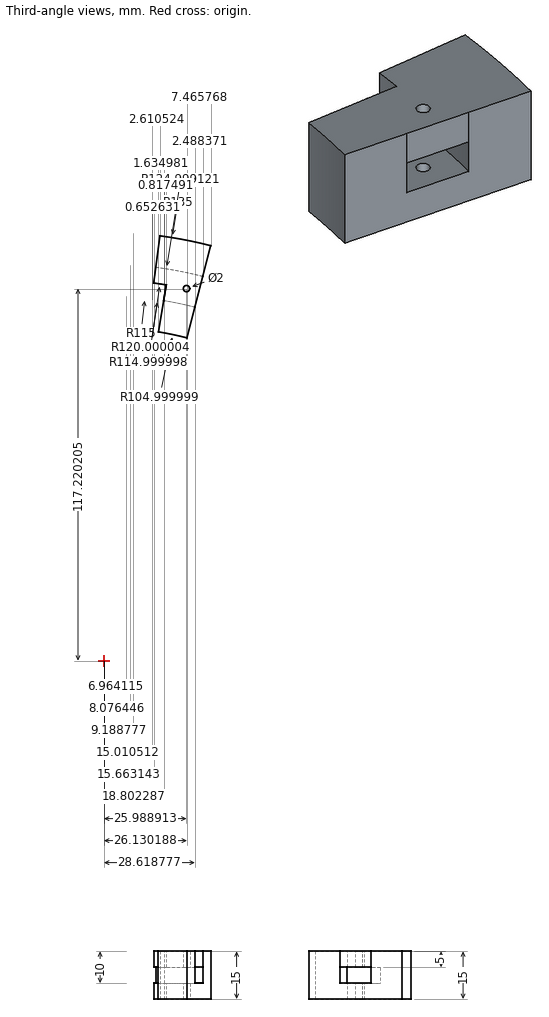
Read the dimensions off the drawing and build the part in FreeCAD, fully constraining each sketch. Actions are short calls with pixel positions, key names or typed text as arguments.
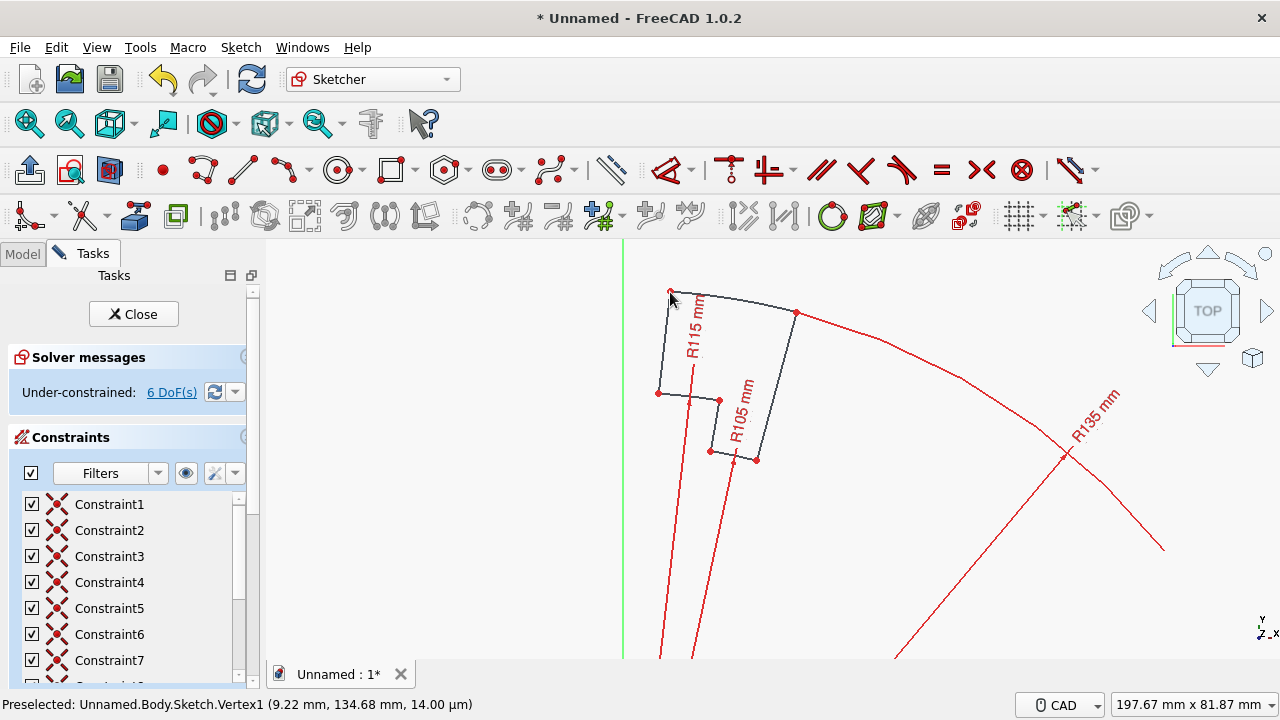
click(670, 292)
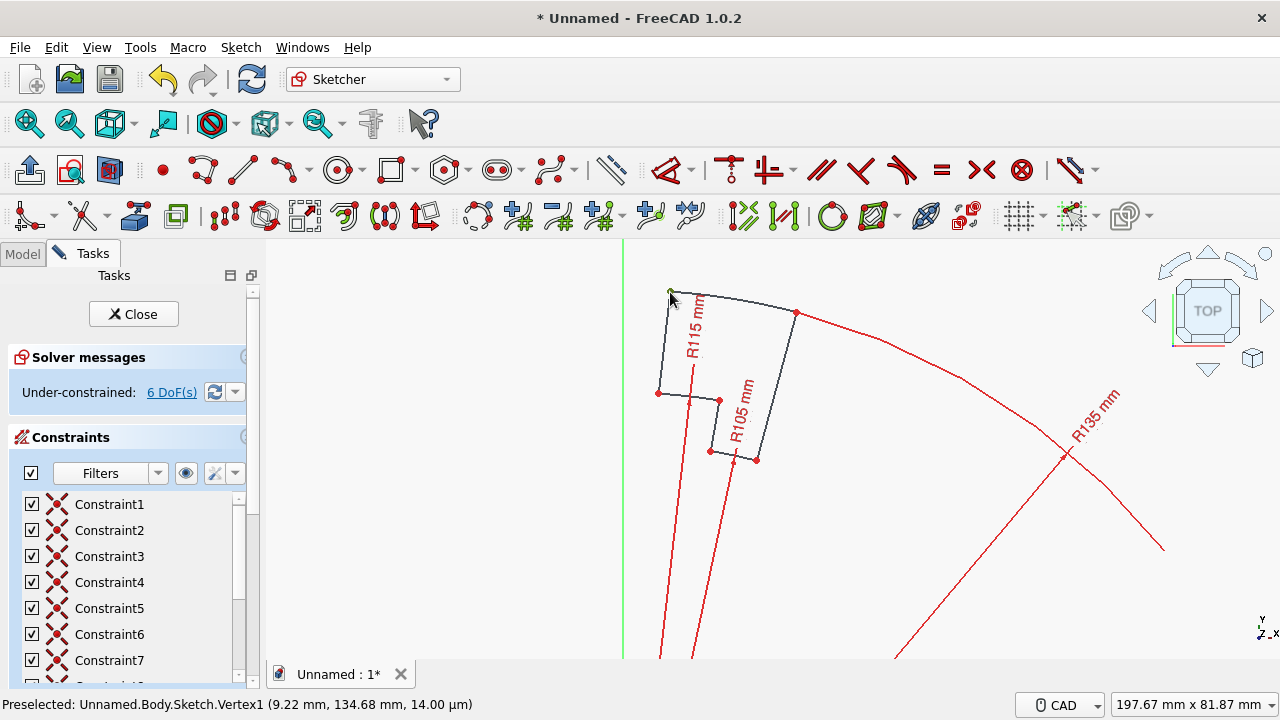
key(l)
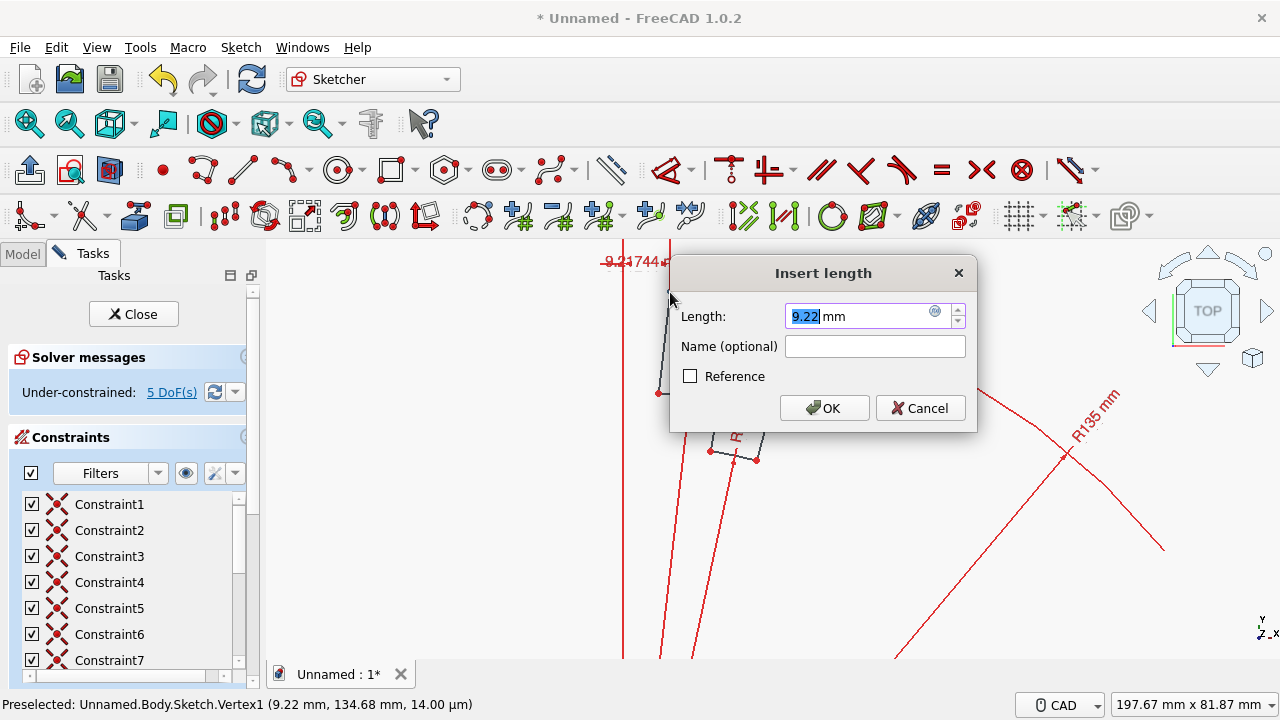
text(9.188777)
key(Return)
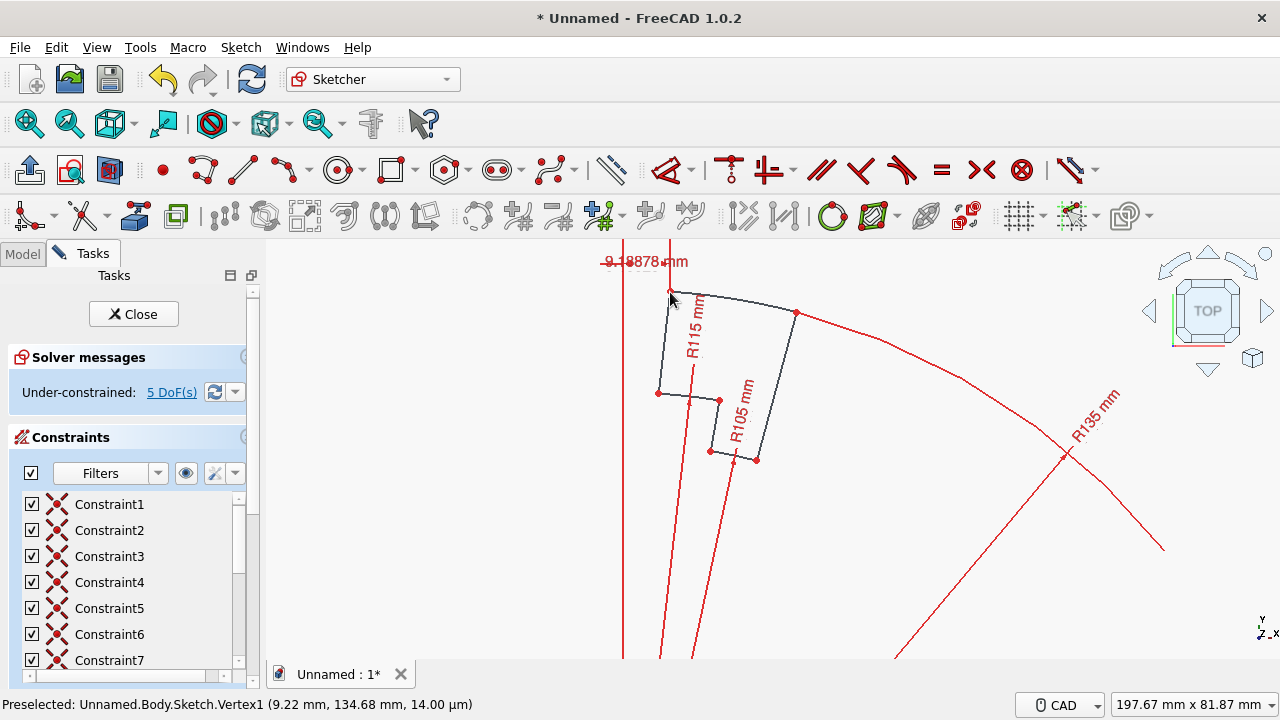
click(659, 394)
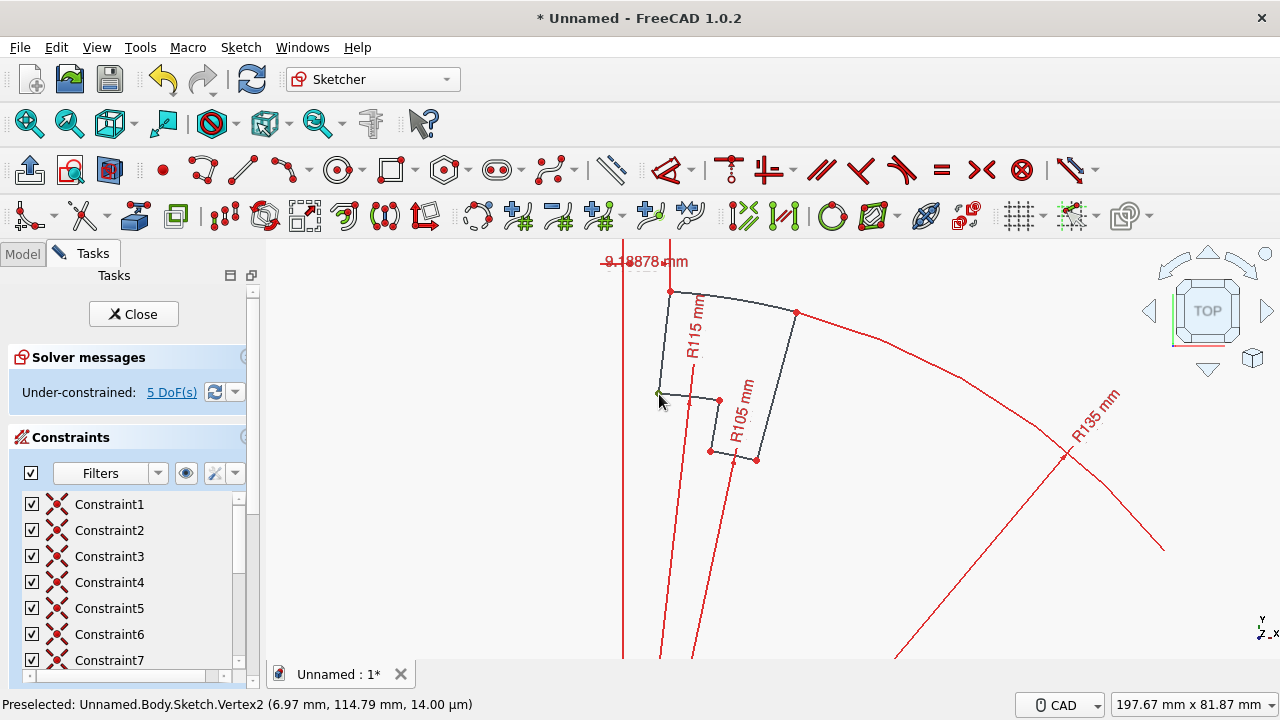
click(694, 170)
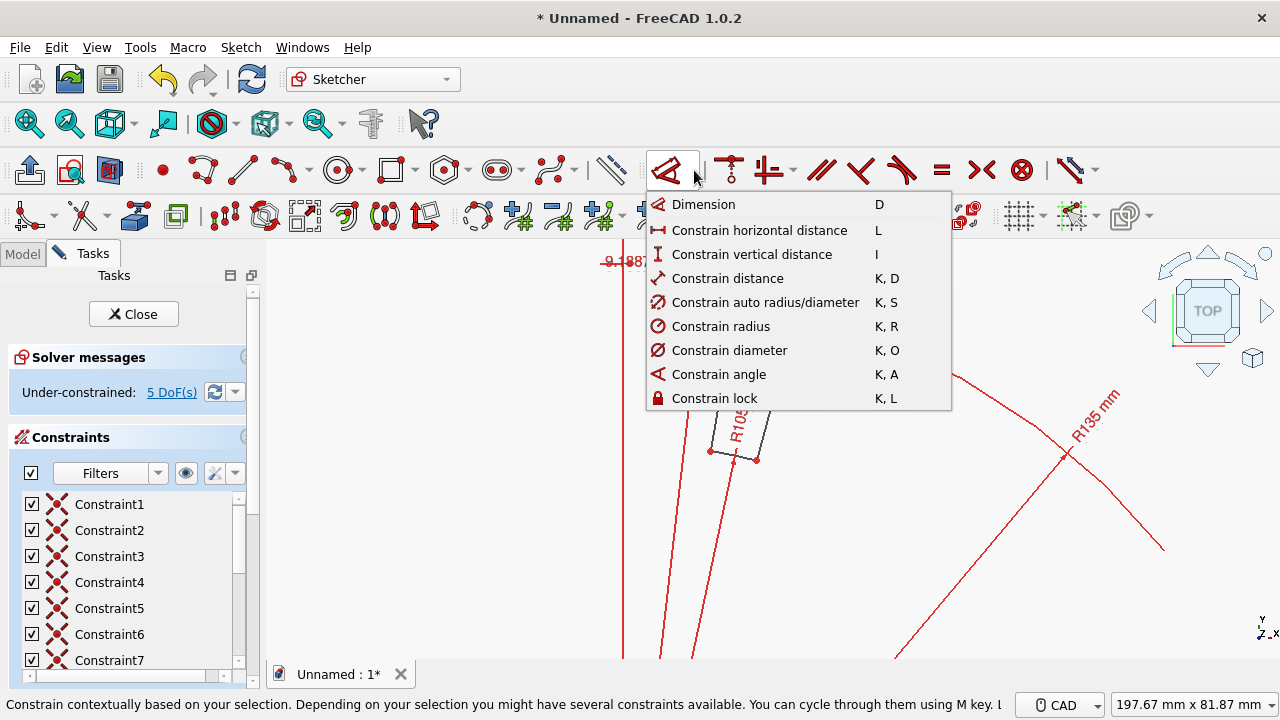
click(799, 230)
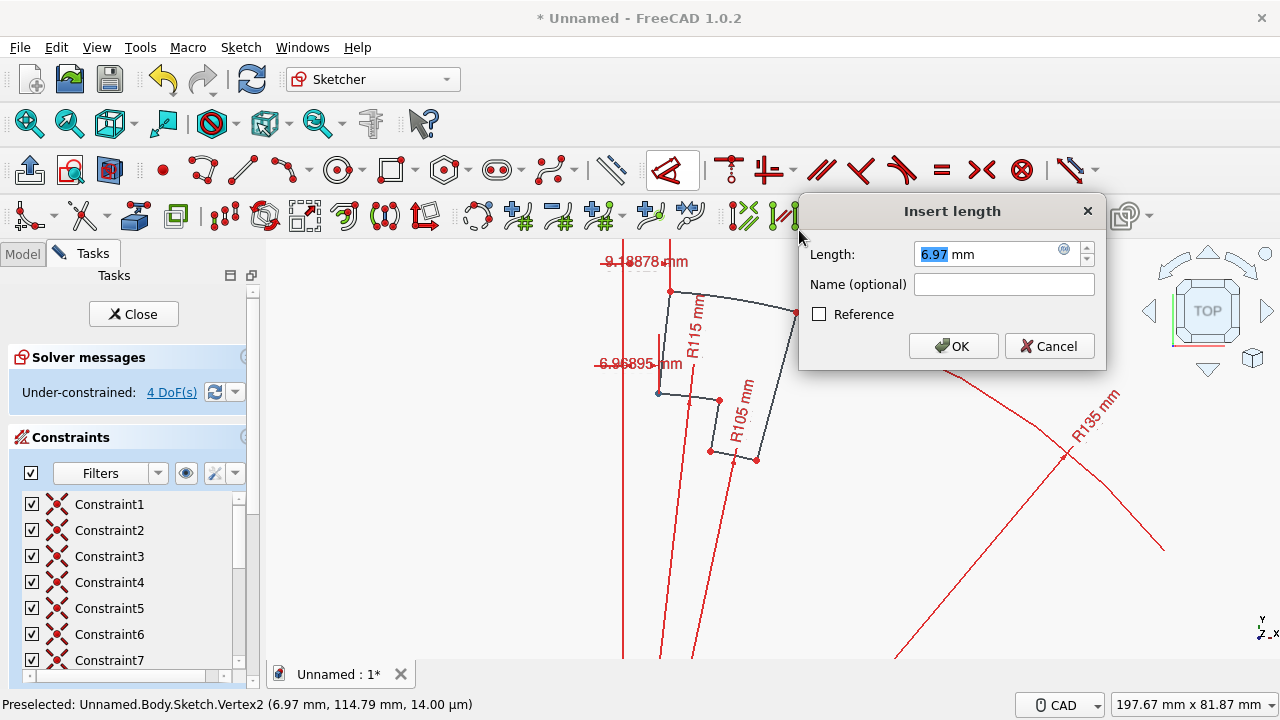
text(6.964115)
key(Return)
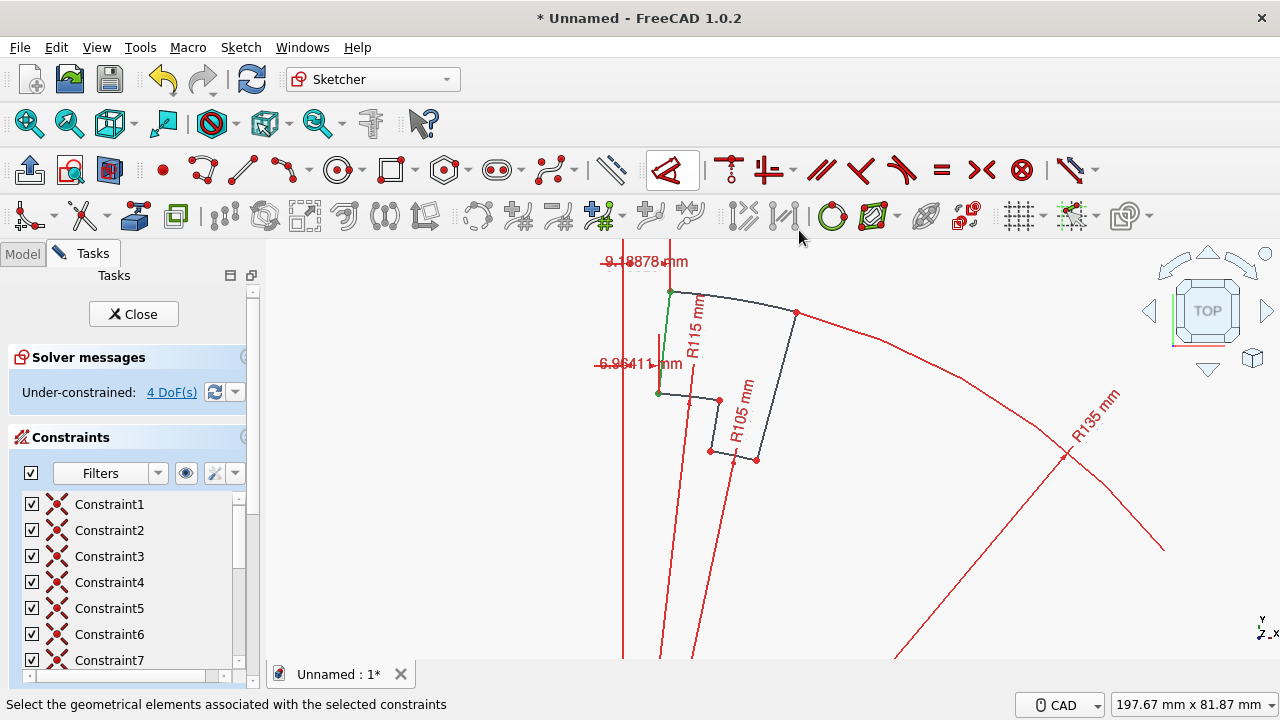
scroll(717, 416, up, 8)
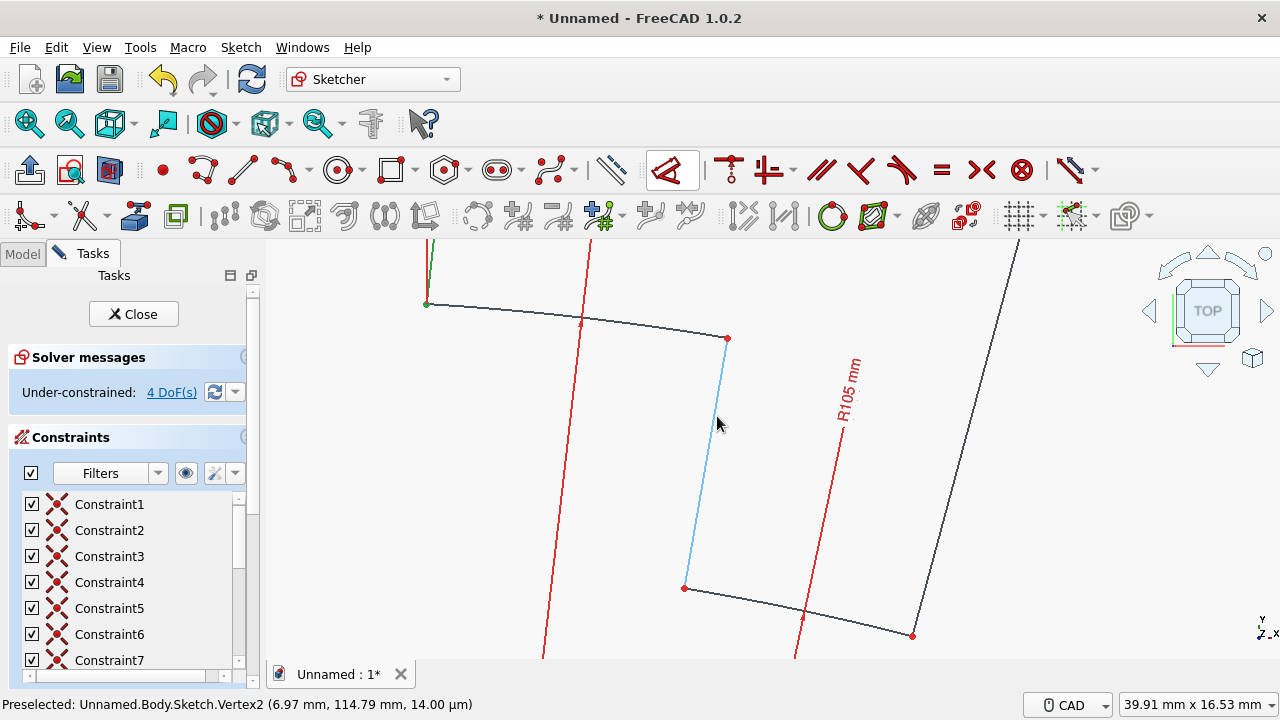
click(715, 413)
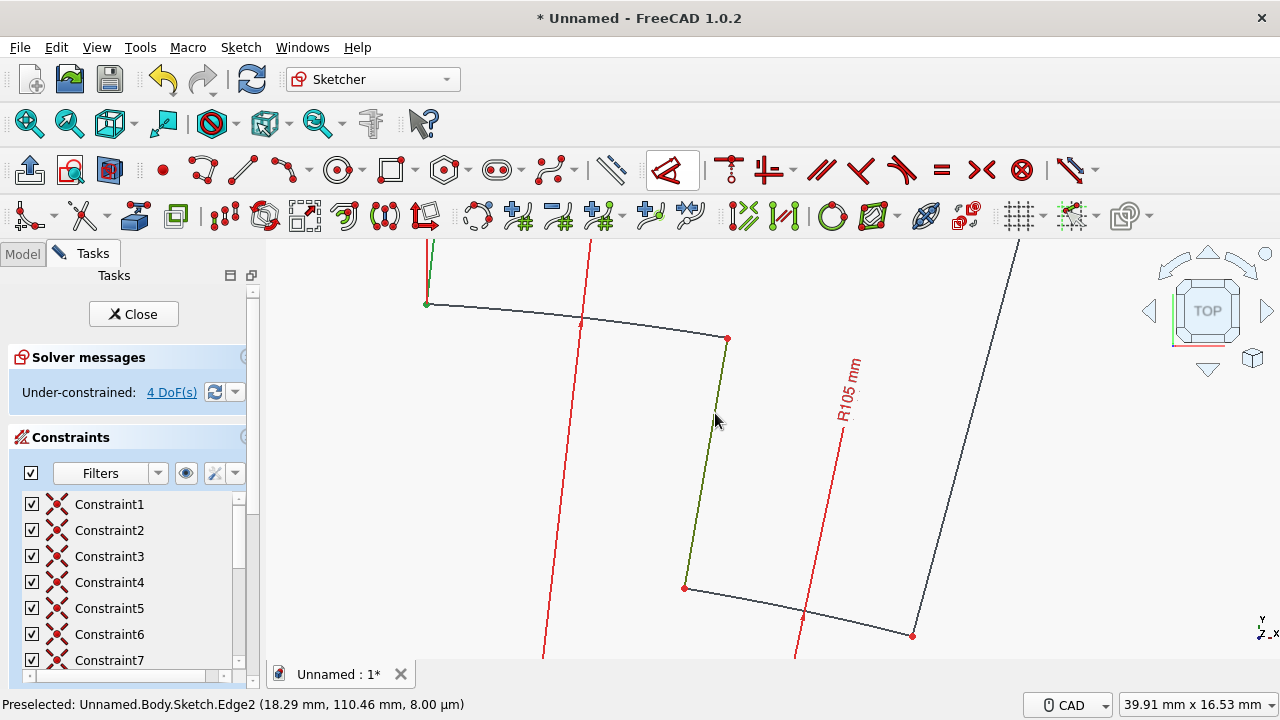
key(l)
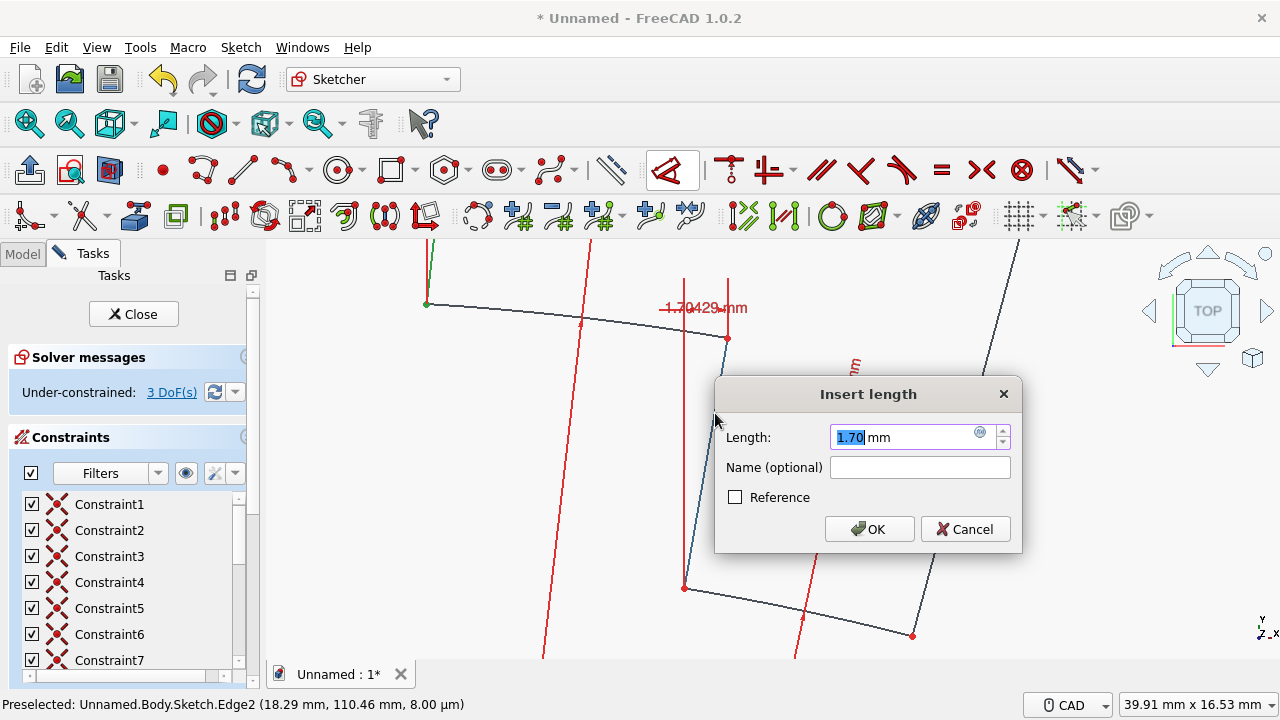
text(1.634981)
key(Return)